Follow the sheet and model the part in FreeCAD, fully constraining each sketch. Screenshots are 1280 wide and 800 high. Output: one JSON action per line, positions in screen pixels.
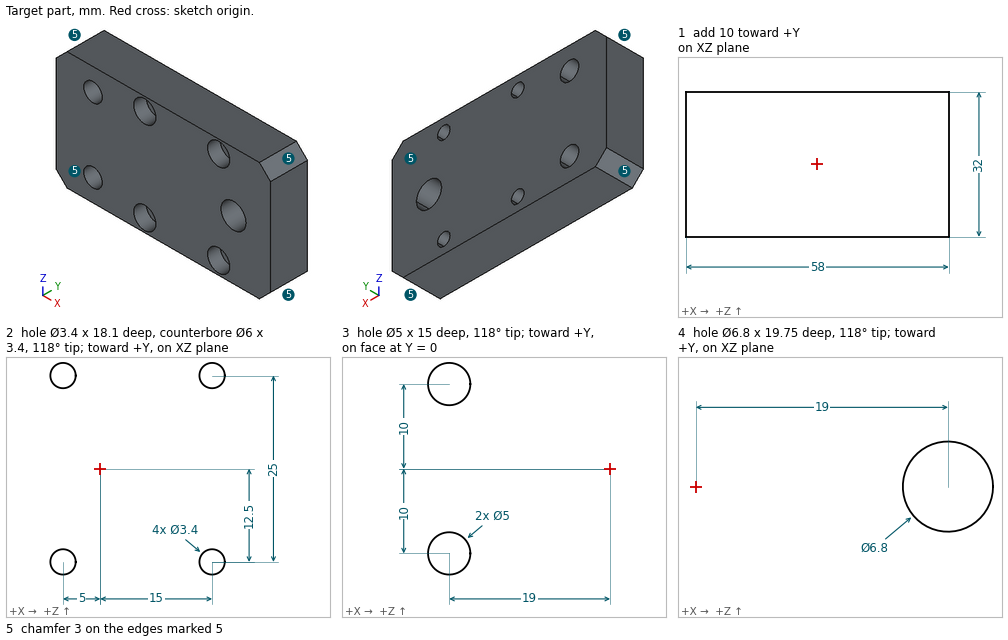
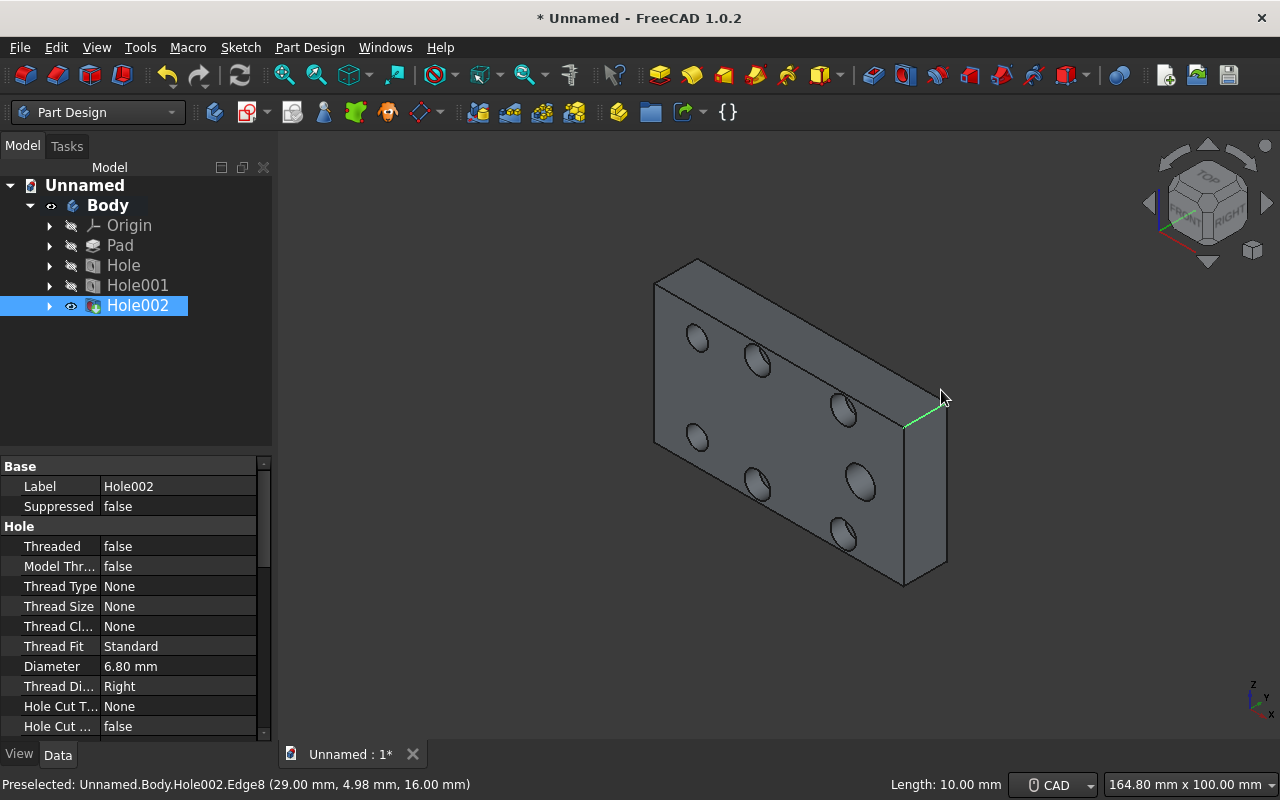
{"action": "key", "text": "2"}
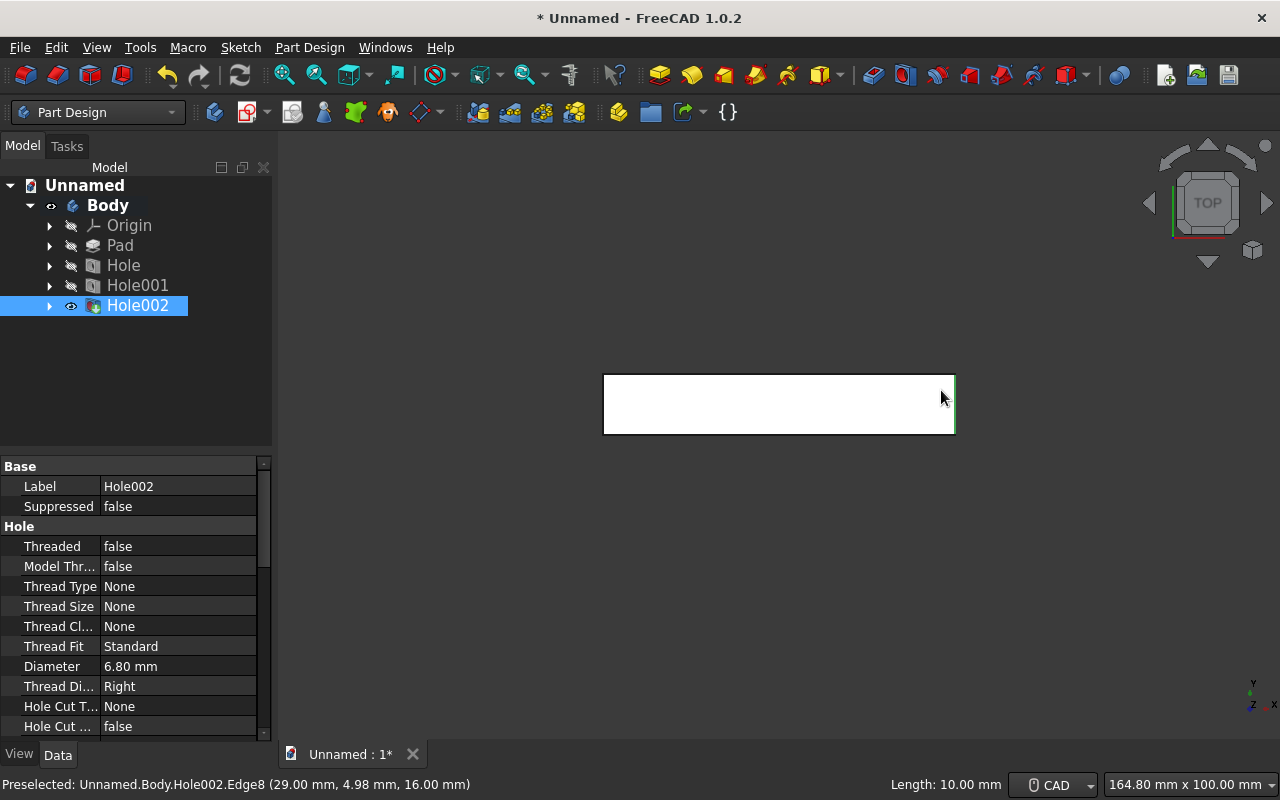
{"action": "left_click", "coordinate": [286, 76]}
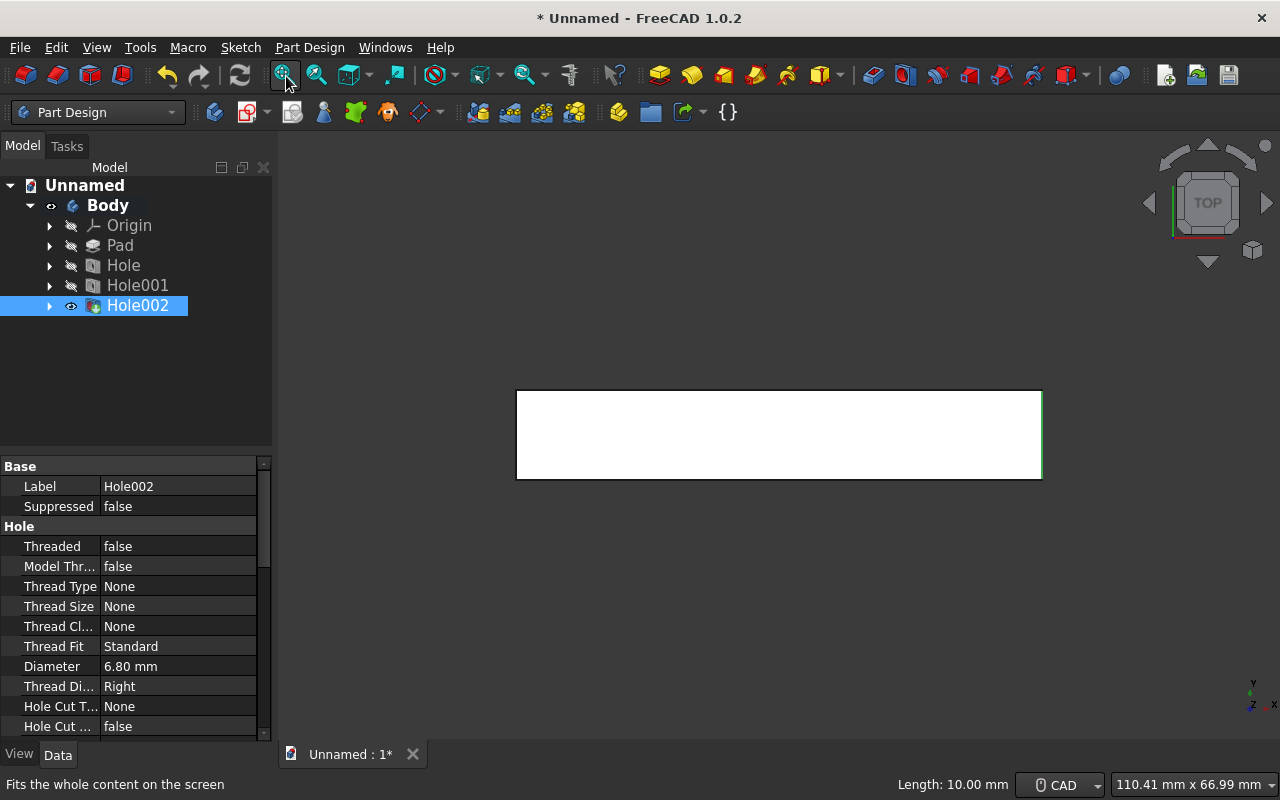
{"action": "left_click", "coordinate": [516, 434], "text": "ctrl"}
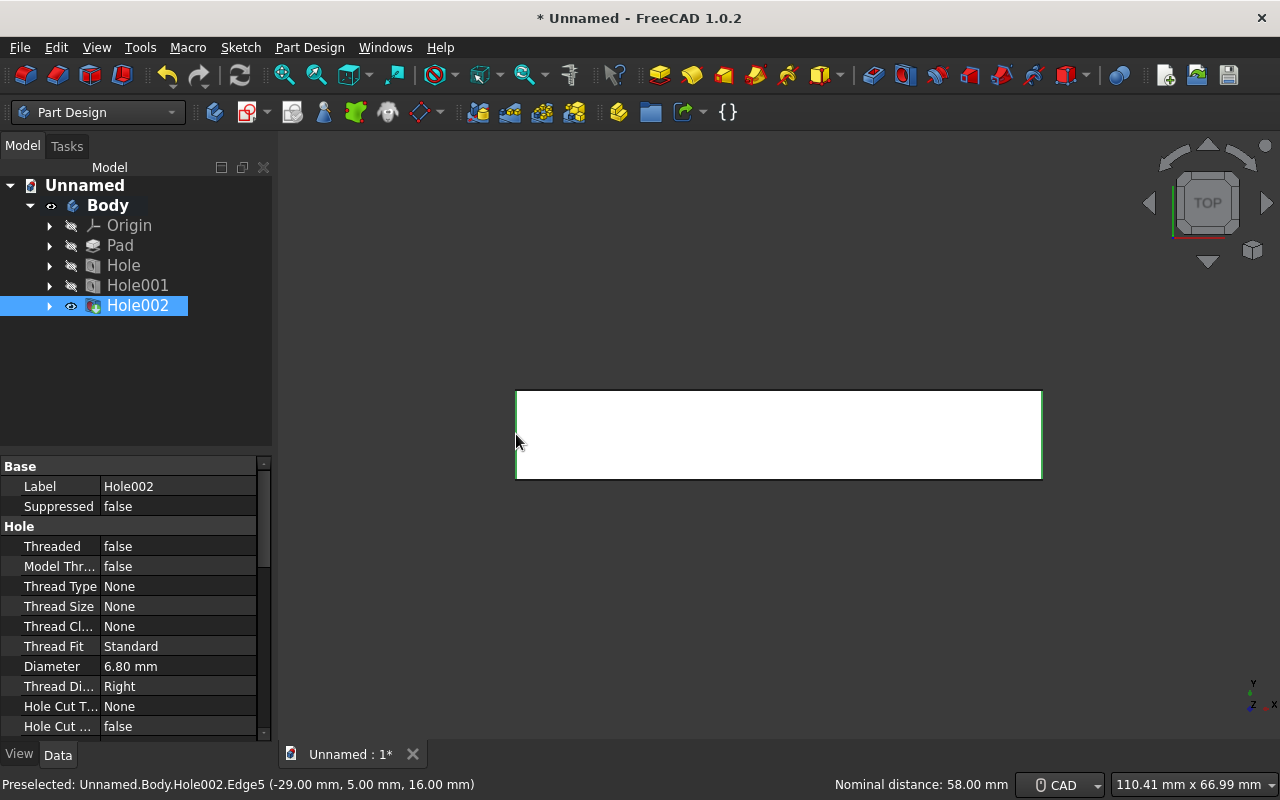
{"action": "key", "text": "1"}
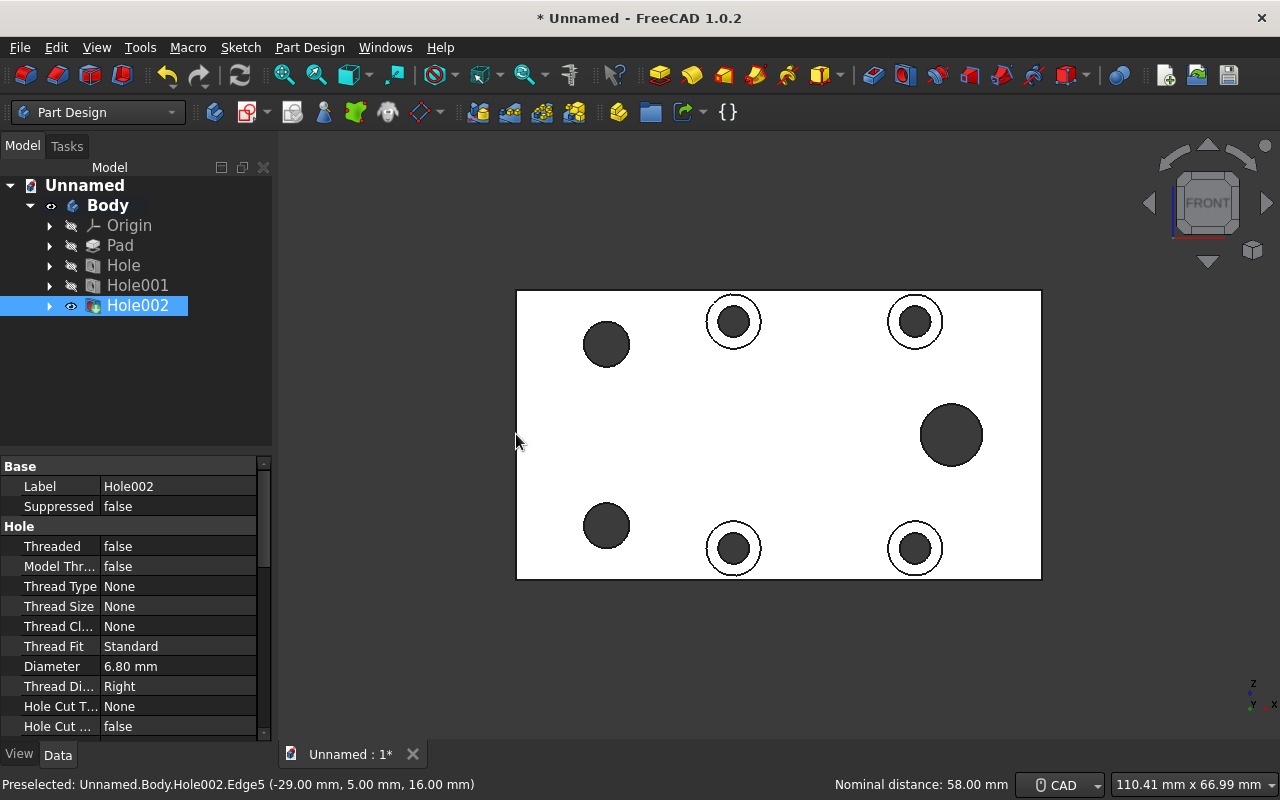
{"action": "key", "text": "3"}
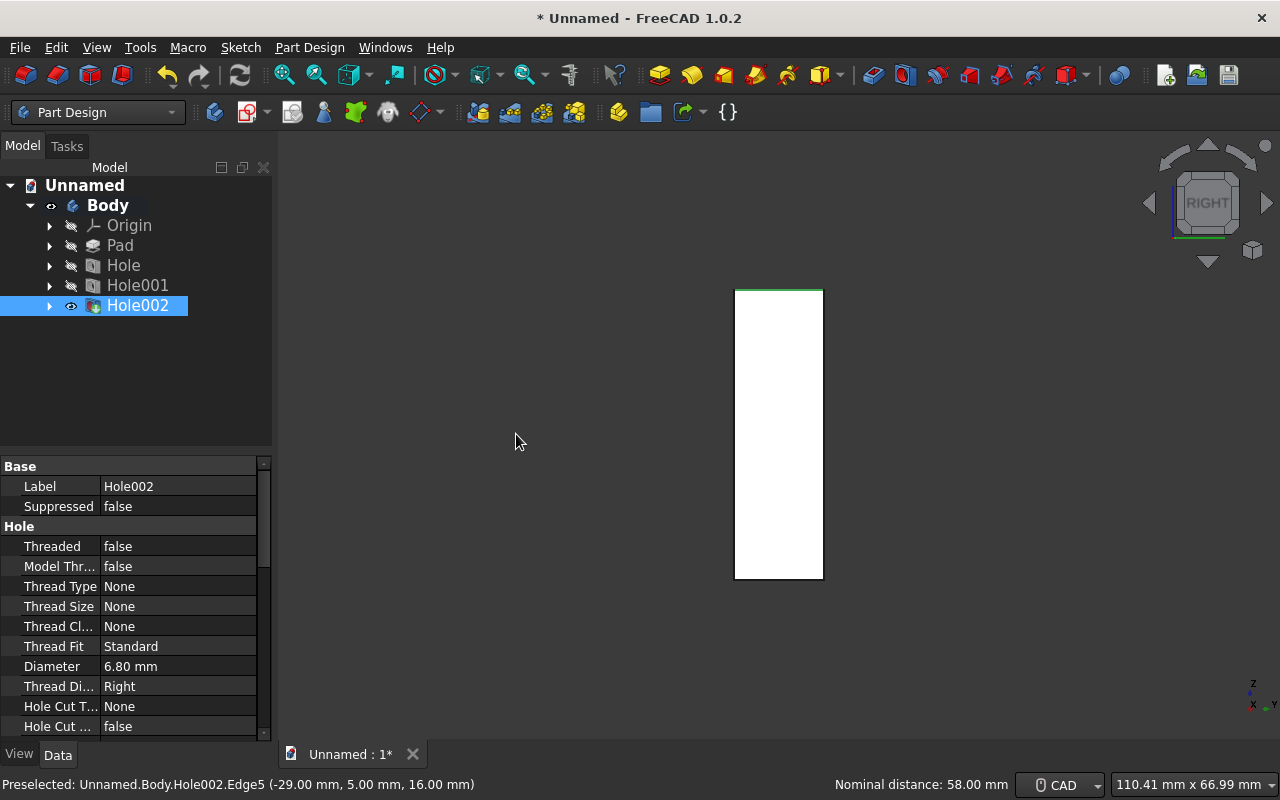
{"action": "left_click", "coordinate": [779, 579], "text": "ctrl"}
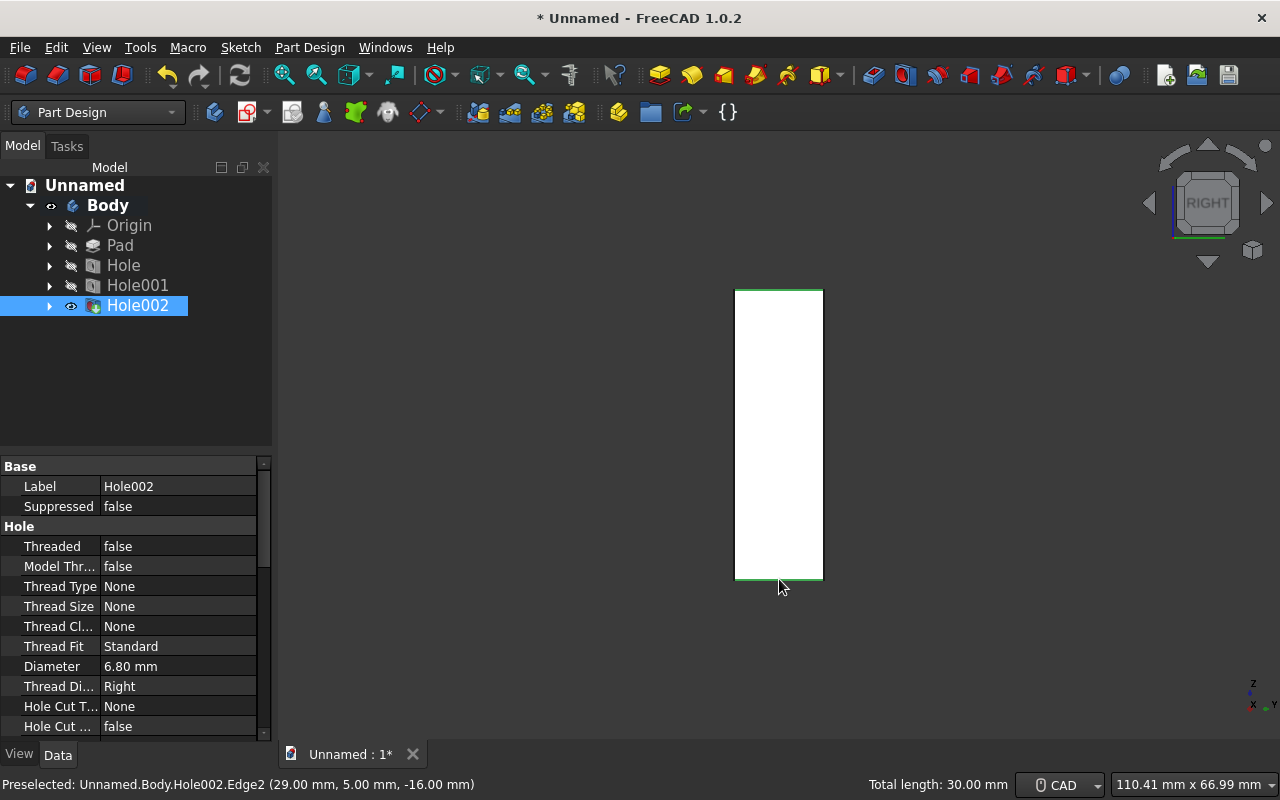
{"action": "key", "text": "5"}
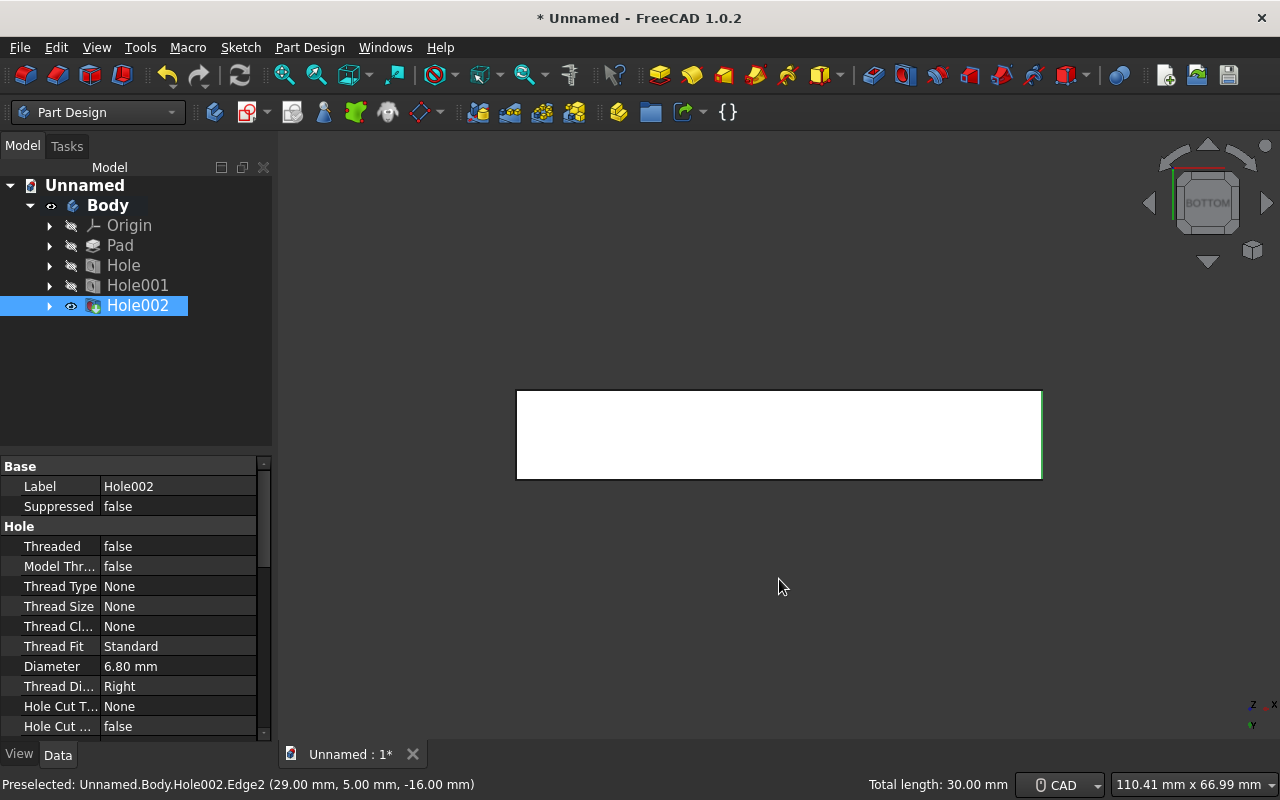
{"action": "left_click", "coordinate": [516, 434], "text": "ctrl"}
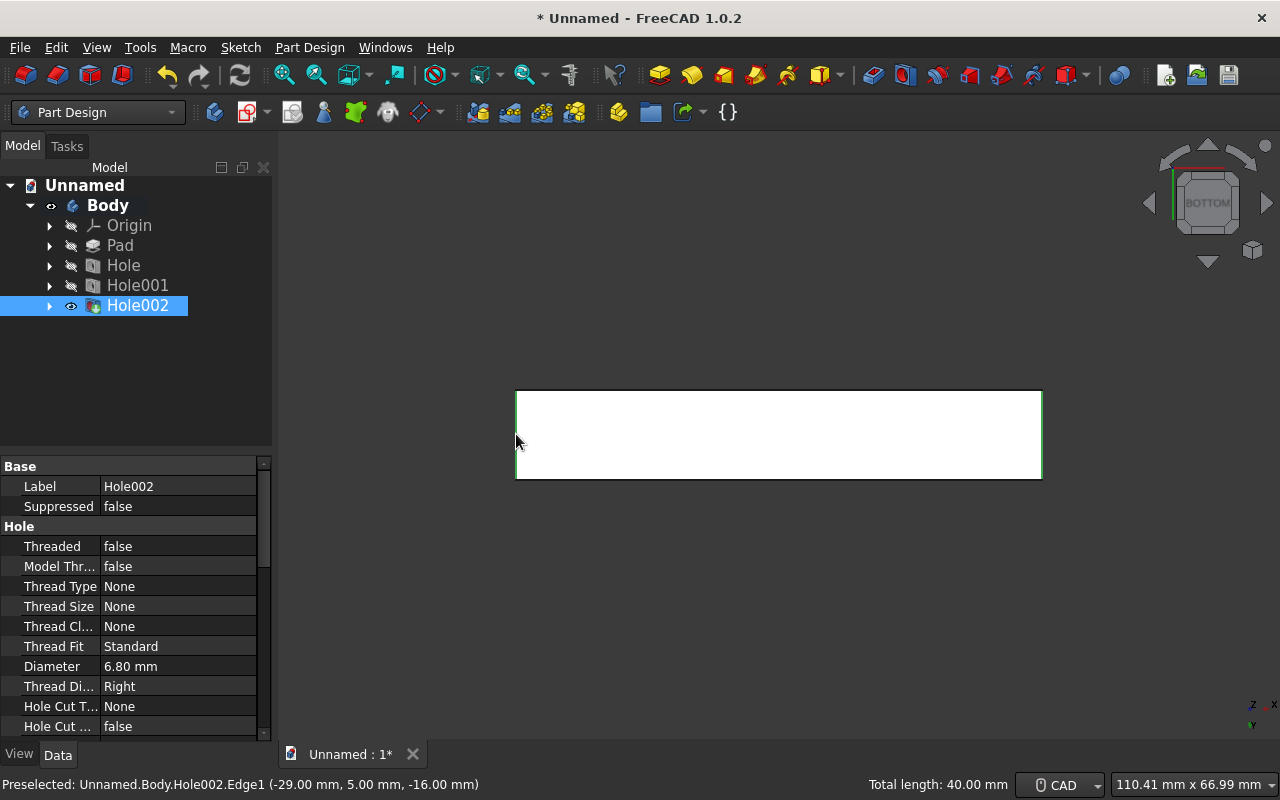
{"action": "left_click", "coordinate": [58, 76]}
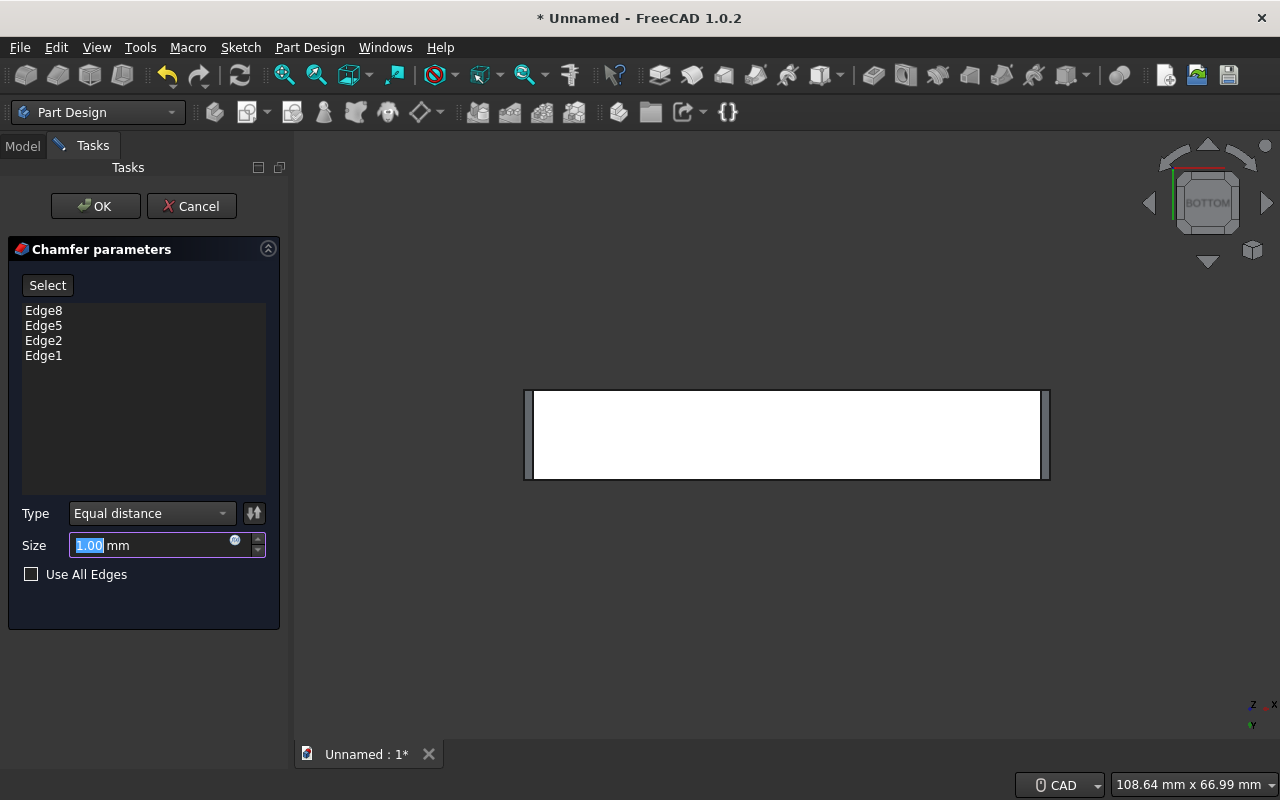
{"action": "type", "text": "3"}
{"action": "key", "text": "Tab"}